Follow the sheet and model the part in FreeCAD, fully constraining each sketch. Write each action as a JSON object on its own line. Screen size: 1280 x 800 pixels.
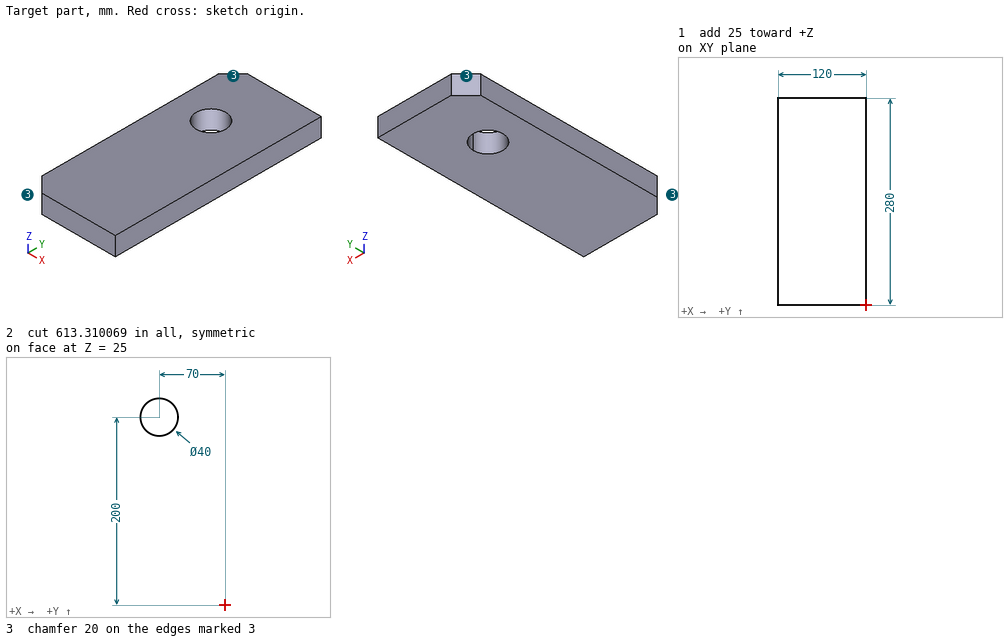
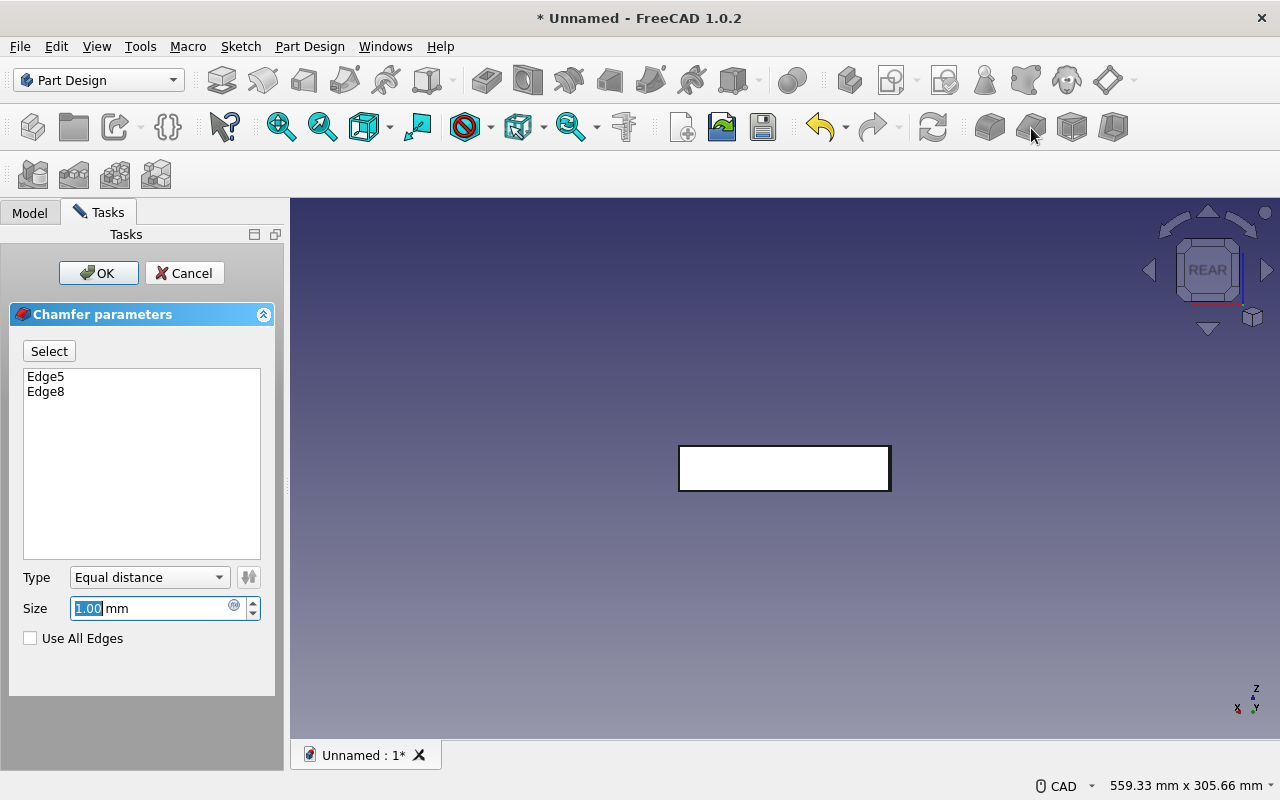
{"action": "type", "text": "20"}
{"action": "key", "text": "Tab"}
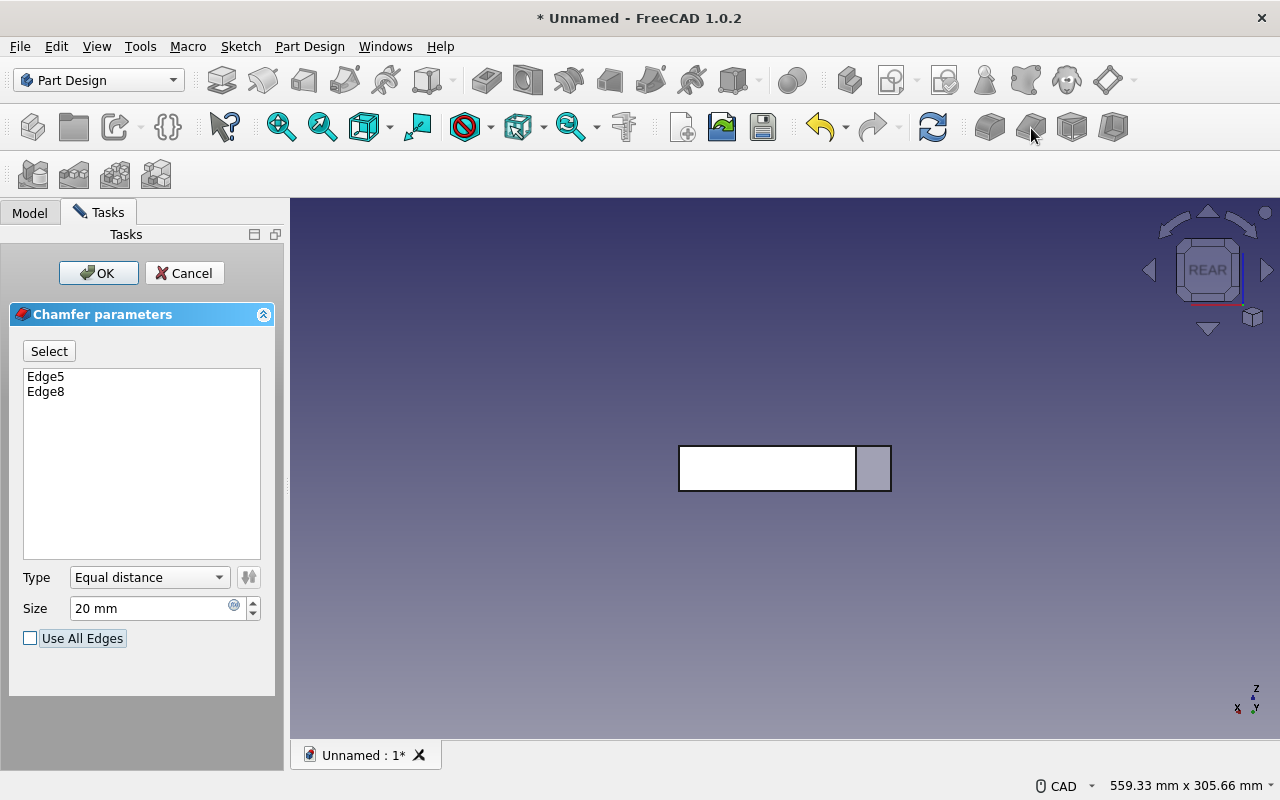
{"action": "left_click", "coordinate": [99, 273]}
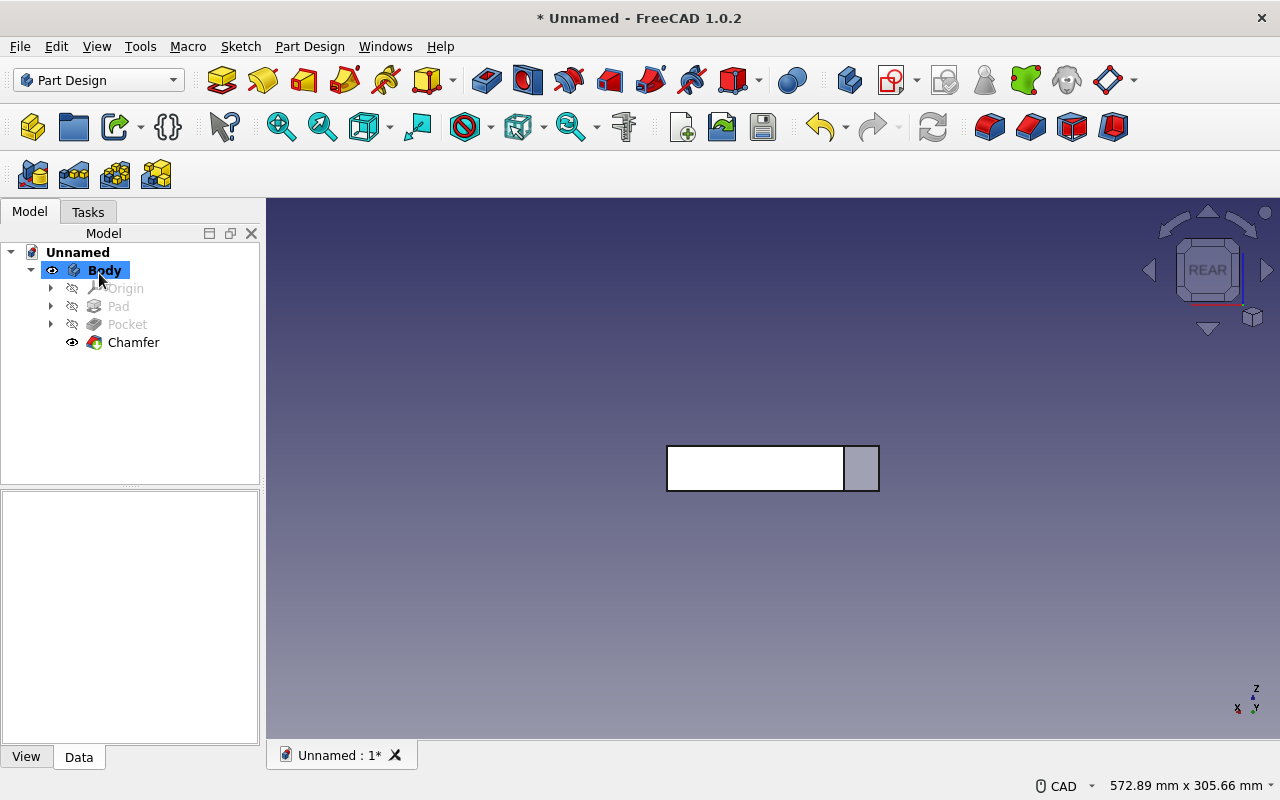
{"action": "key", "text": "0"}